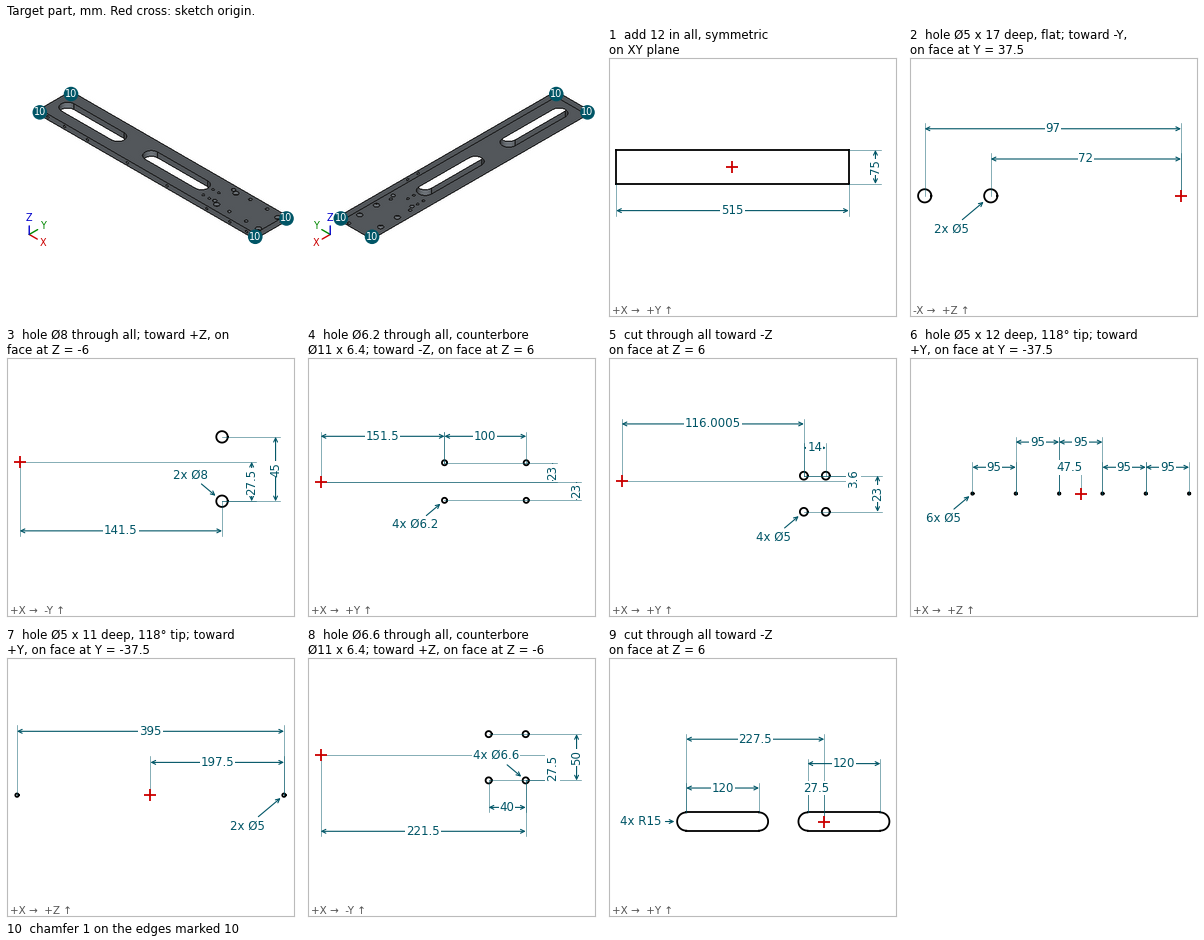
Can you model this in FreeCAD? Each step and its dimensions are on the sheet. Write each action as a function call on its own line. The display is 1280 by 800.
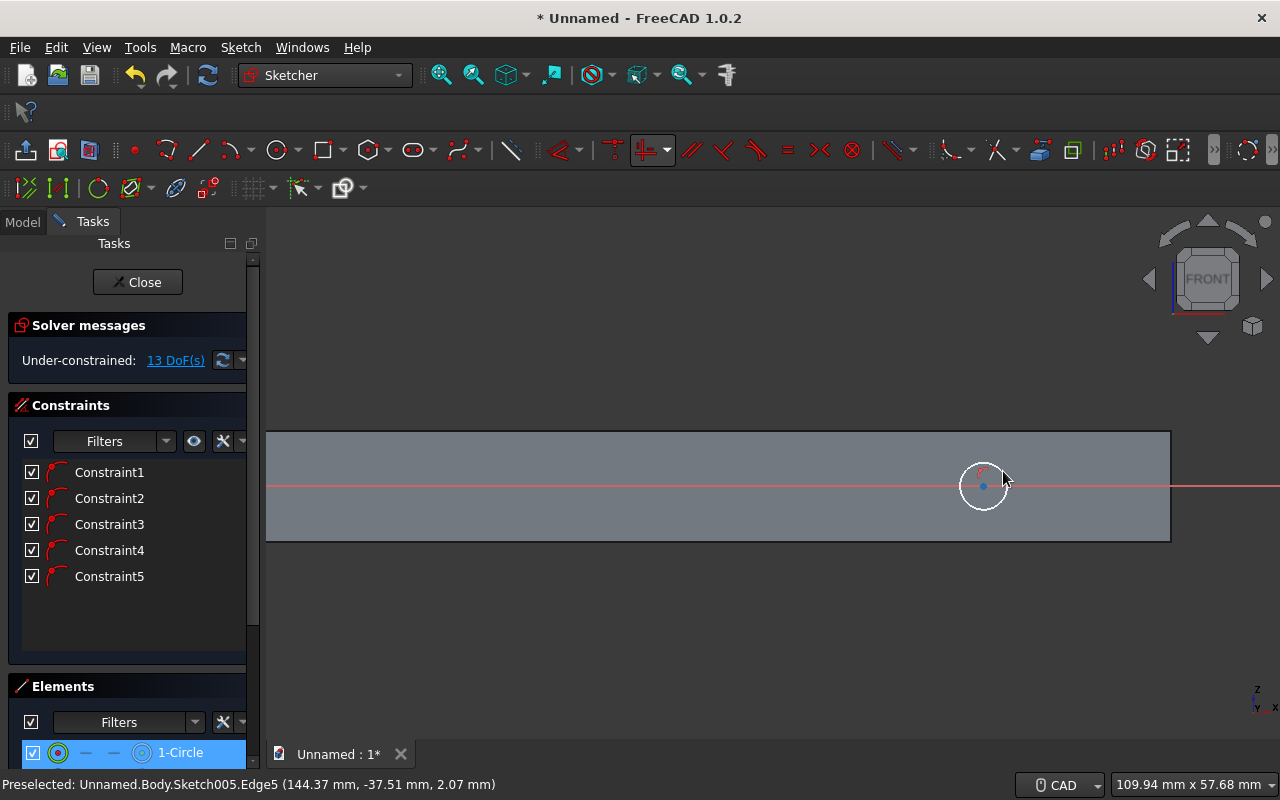
click(1000, 470)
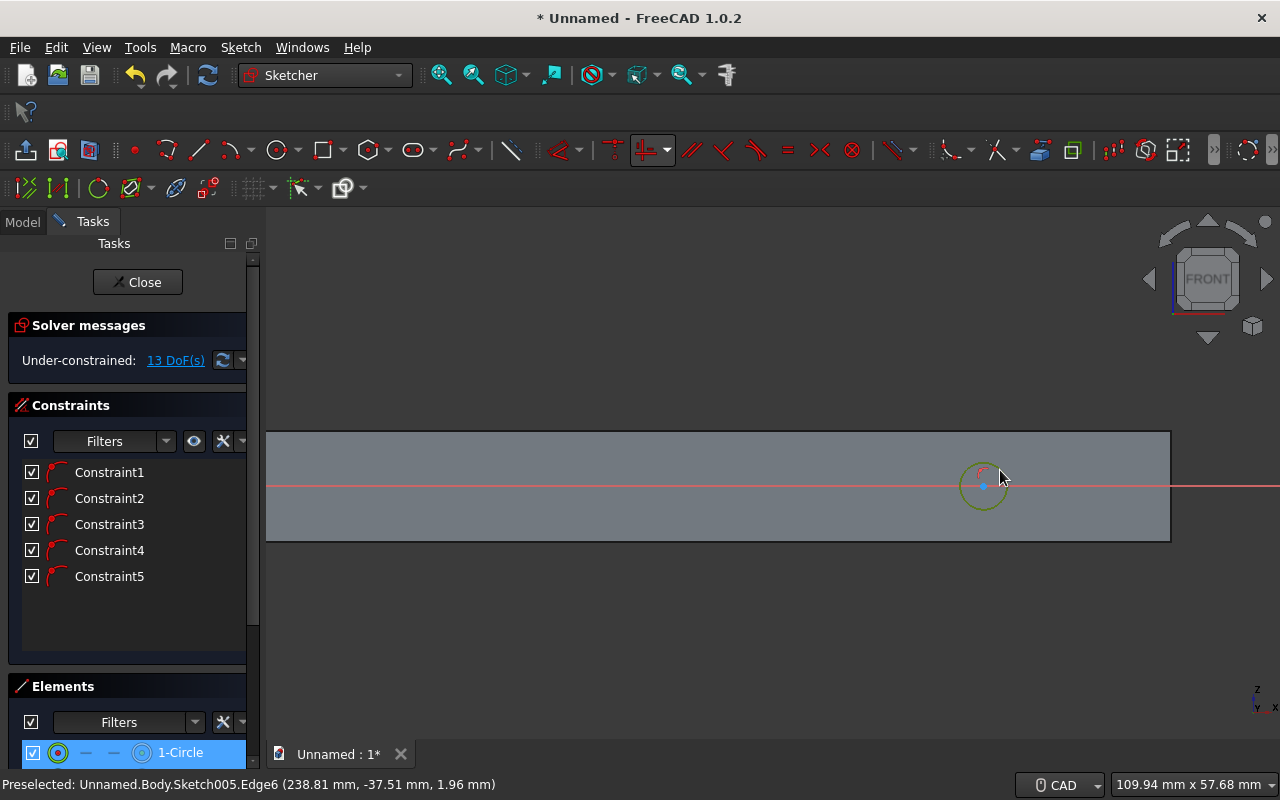
click(788, 150)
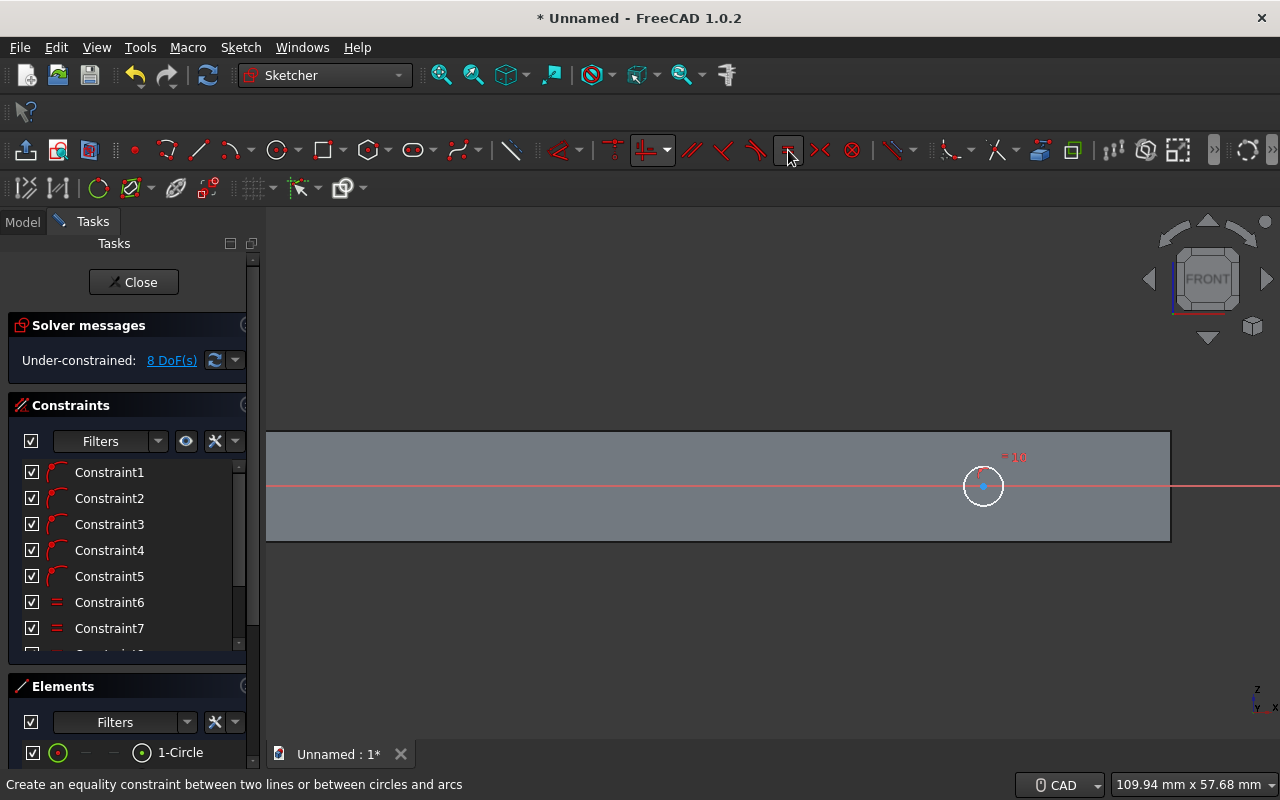
scroll(1003, 471, down, 10)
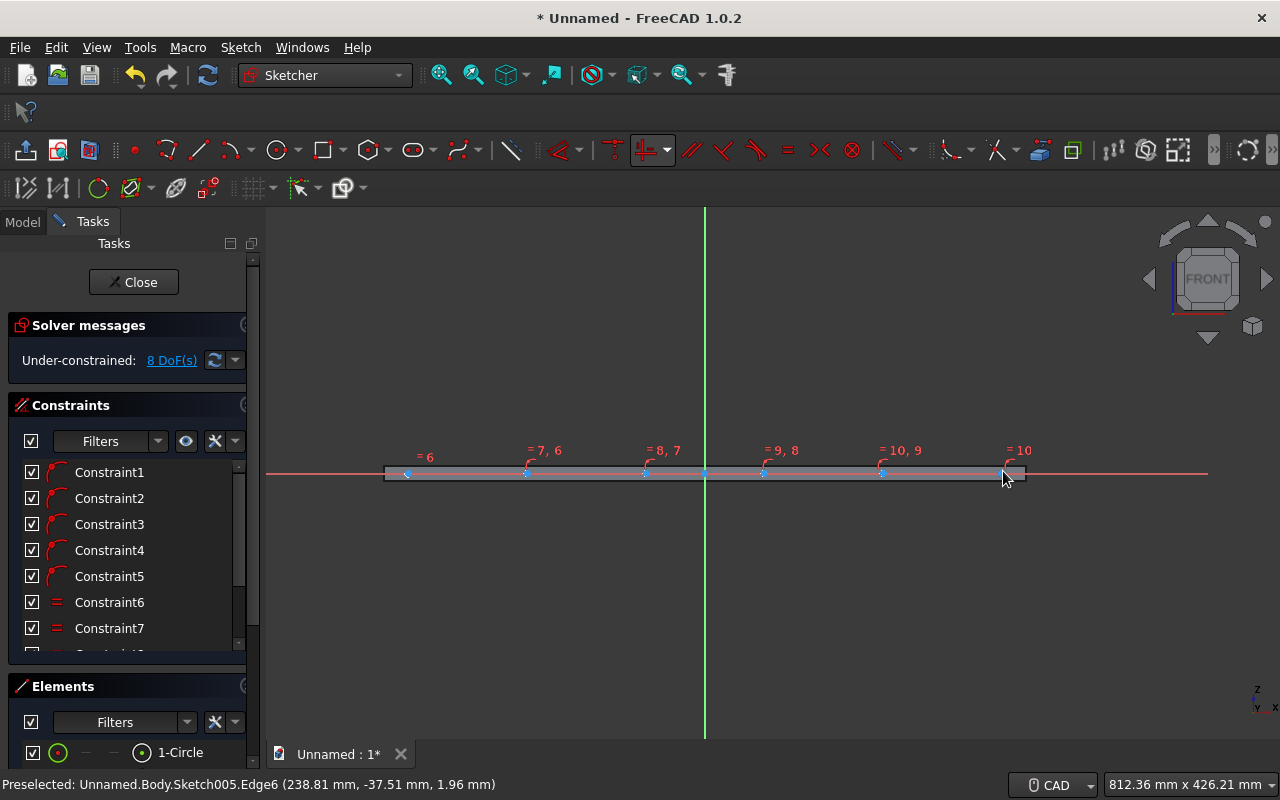
click(408, 474)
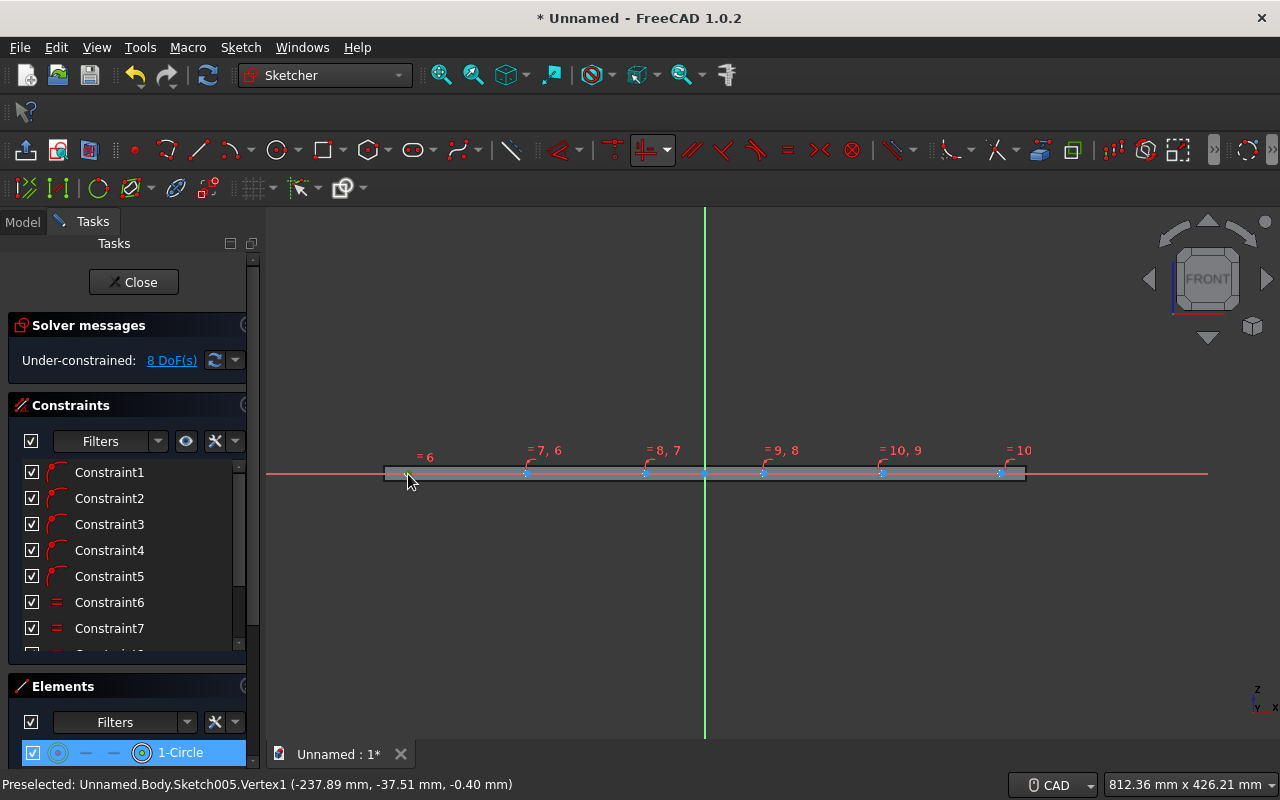
click(353, 473)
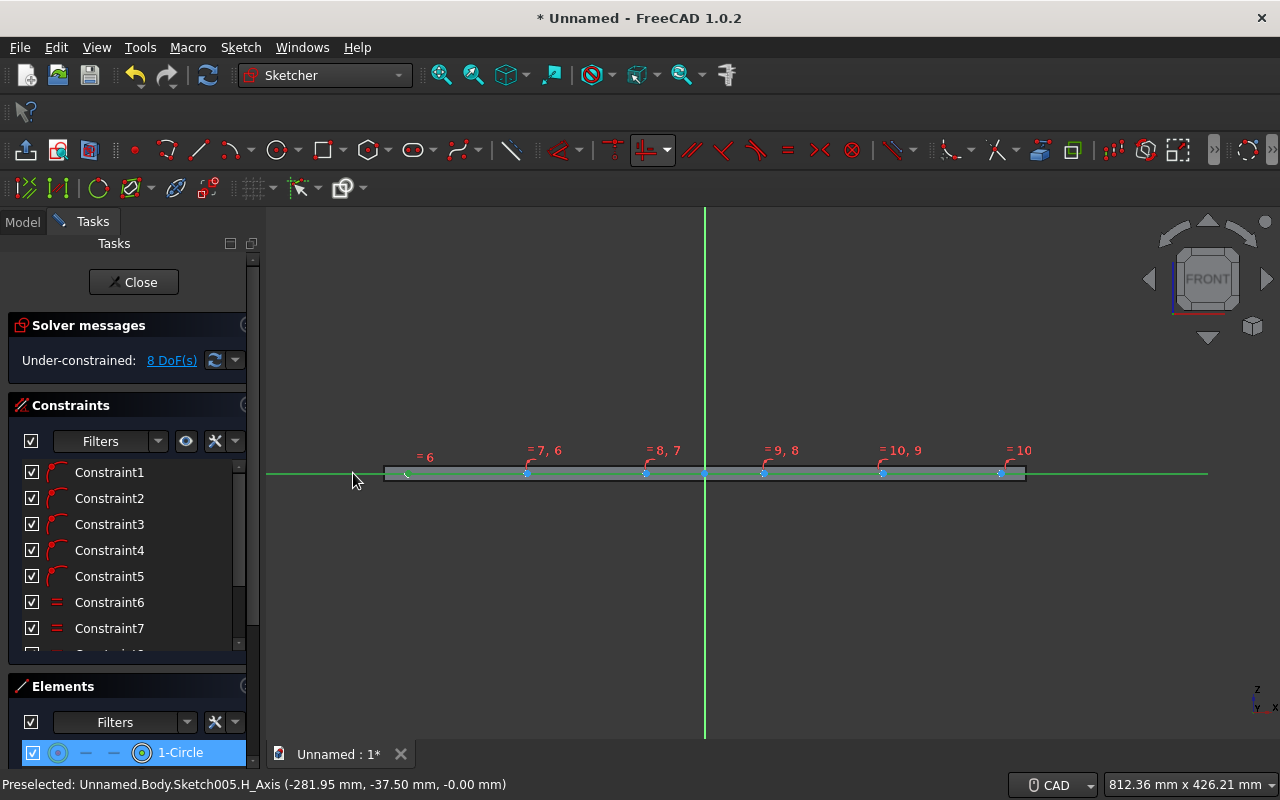
key(c)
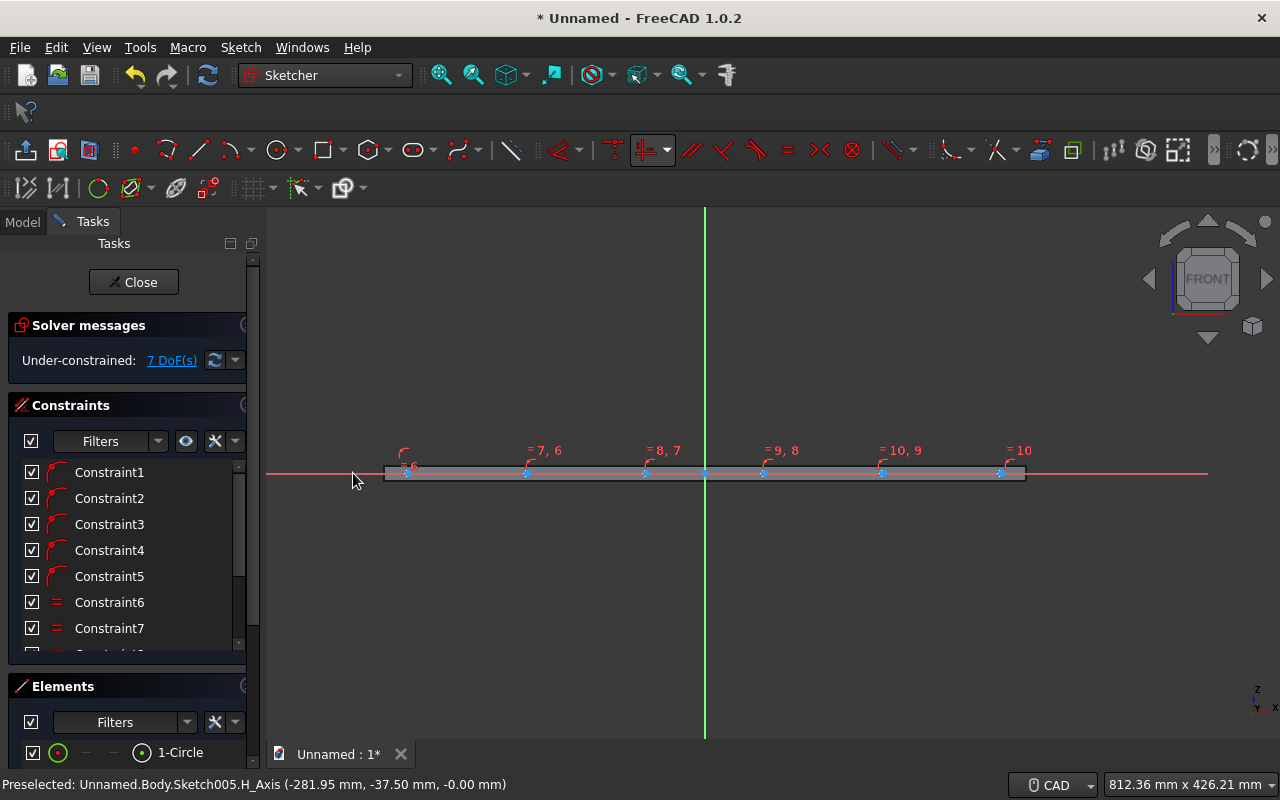
click(558, 150)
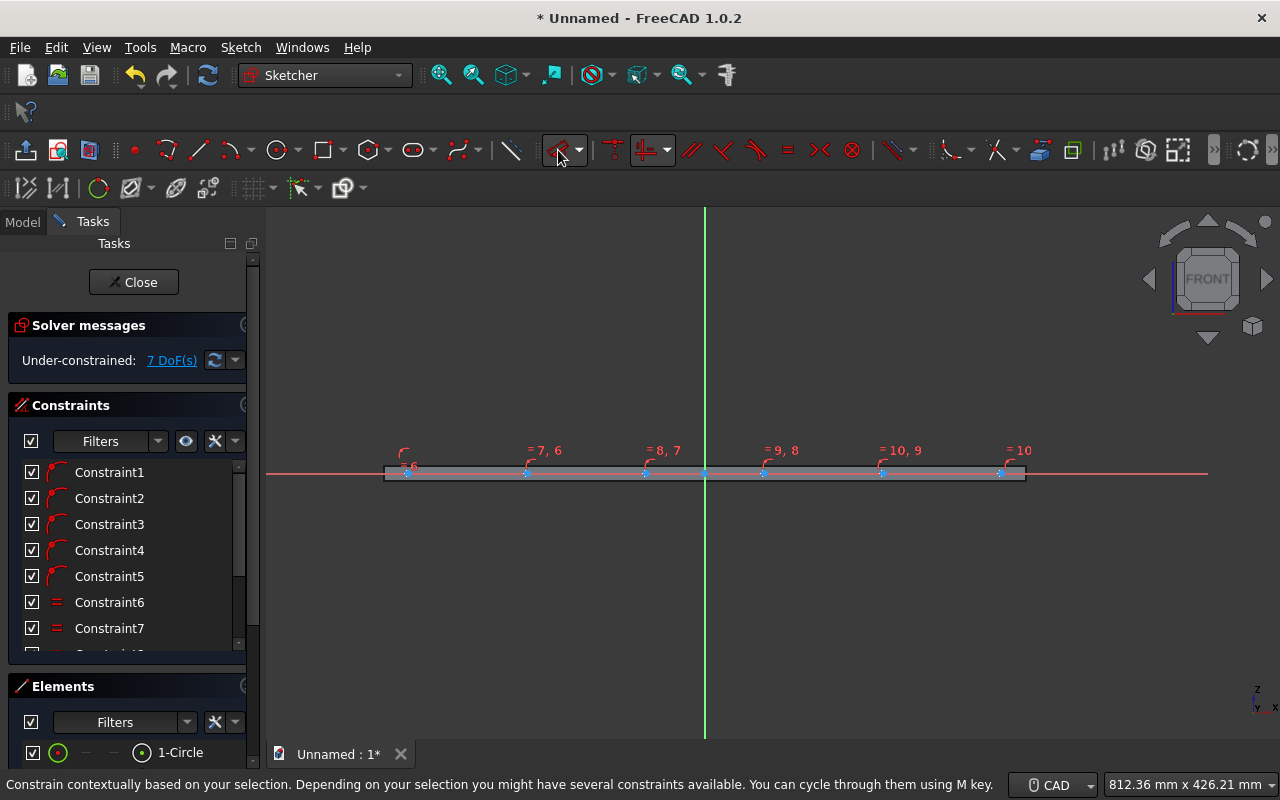
scroll(410, 475, up, 10)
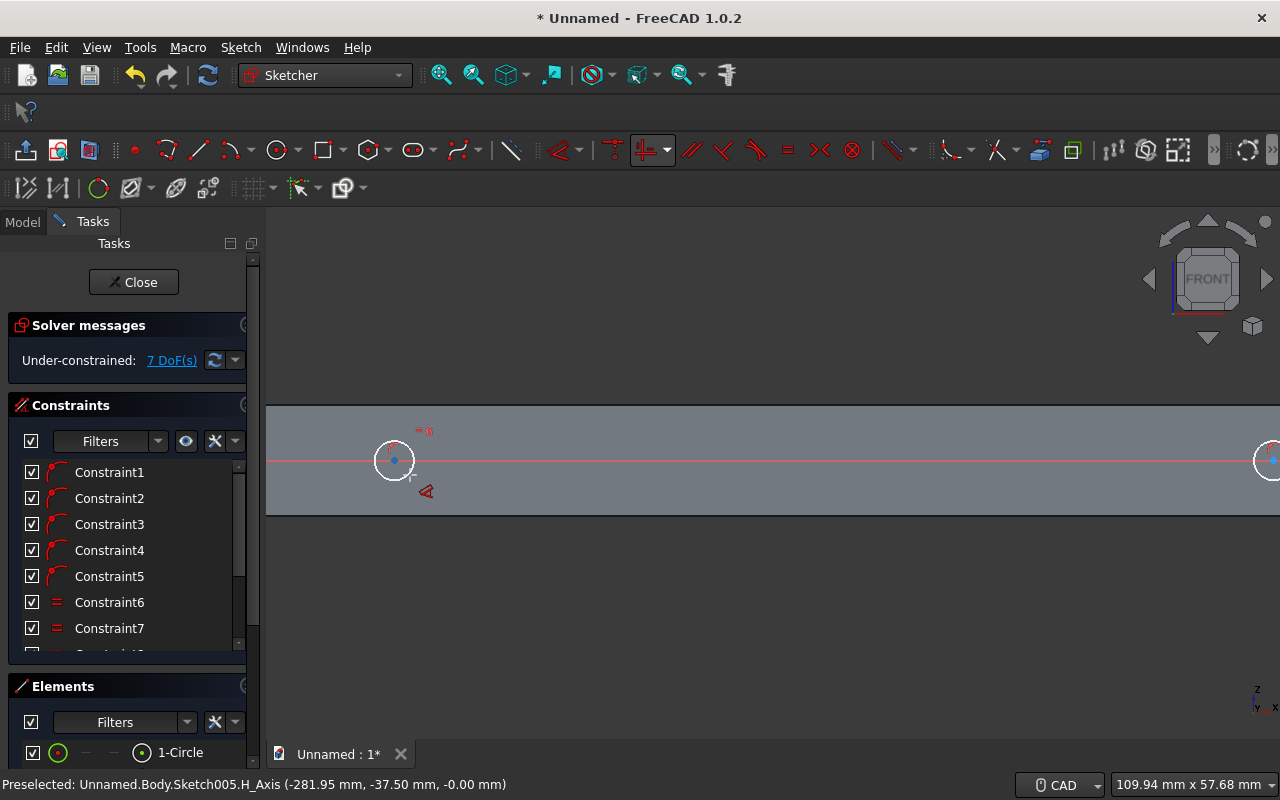
click(408, 474)
click(431, 496)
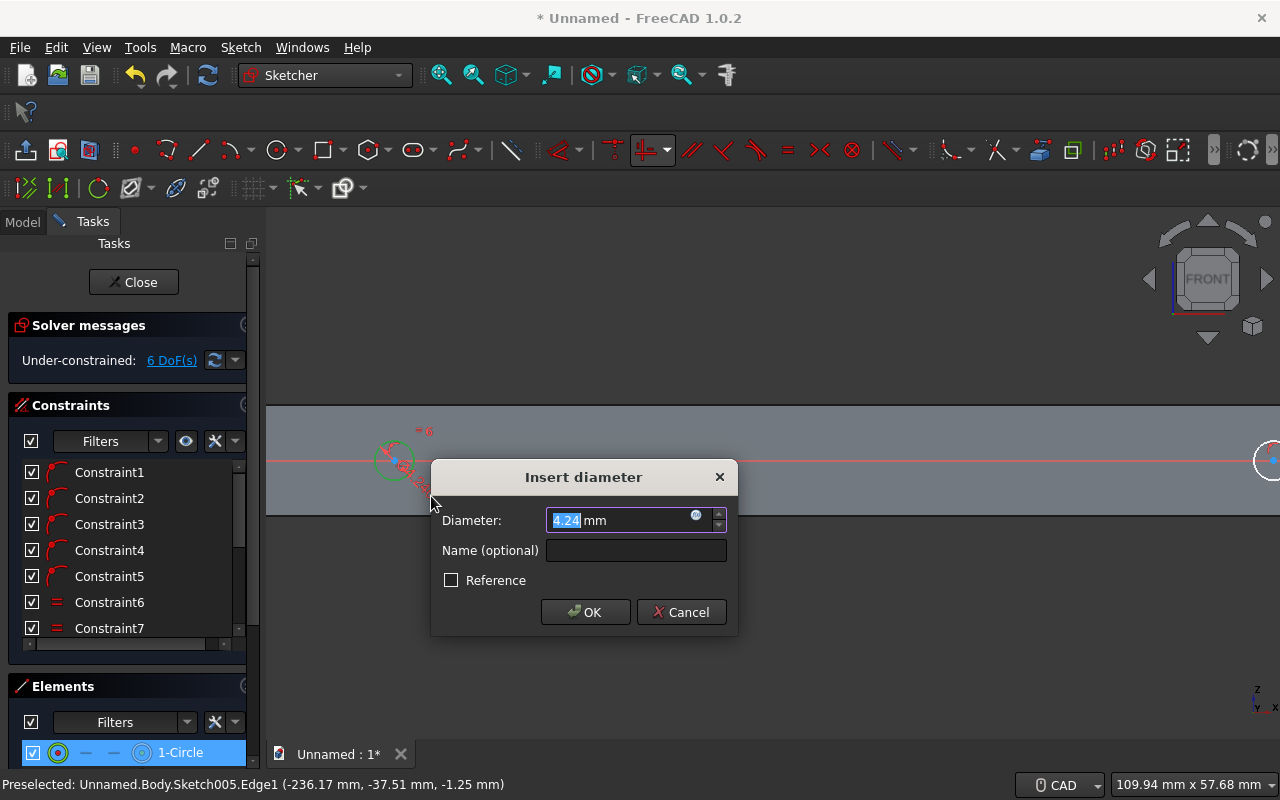
text(5)
key(Return)